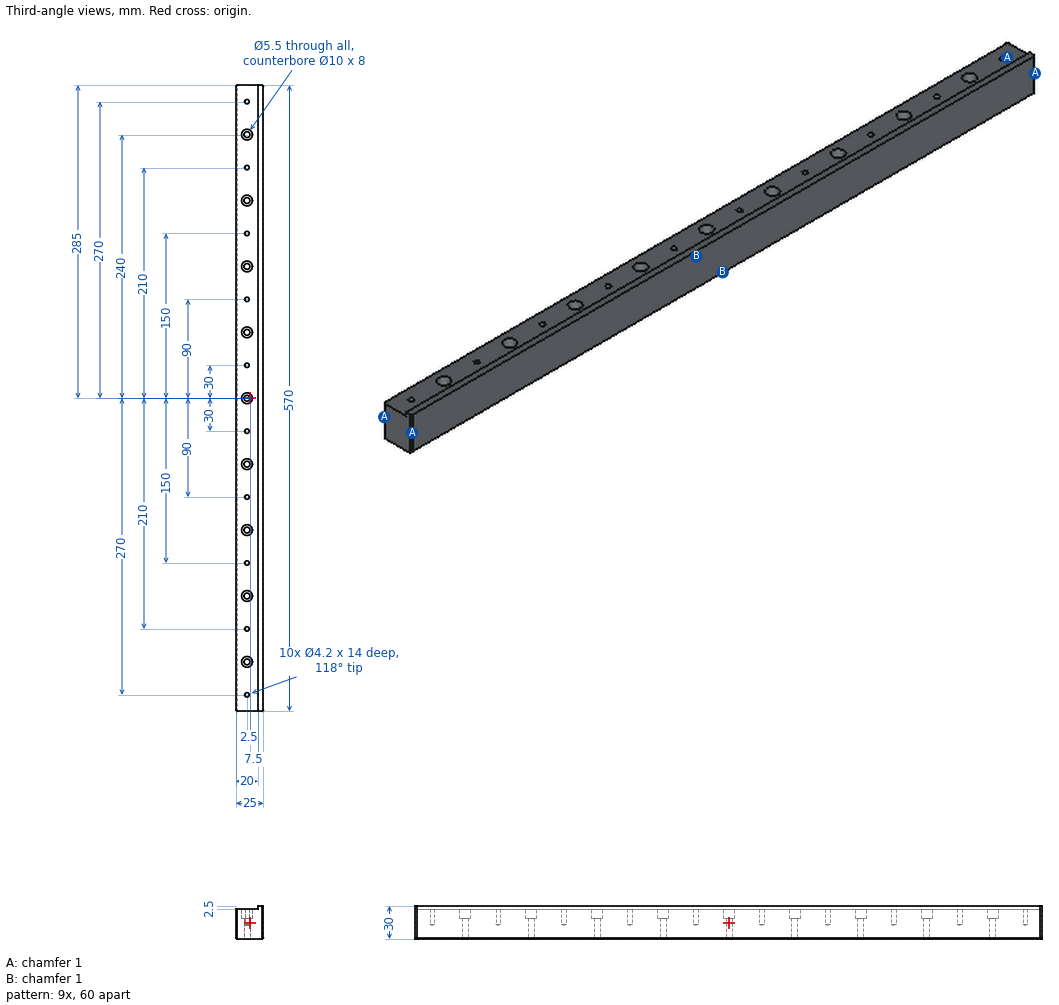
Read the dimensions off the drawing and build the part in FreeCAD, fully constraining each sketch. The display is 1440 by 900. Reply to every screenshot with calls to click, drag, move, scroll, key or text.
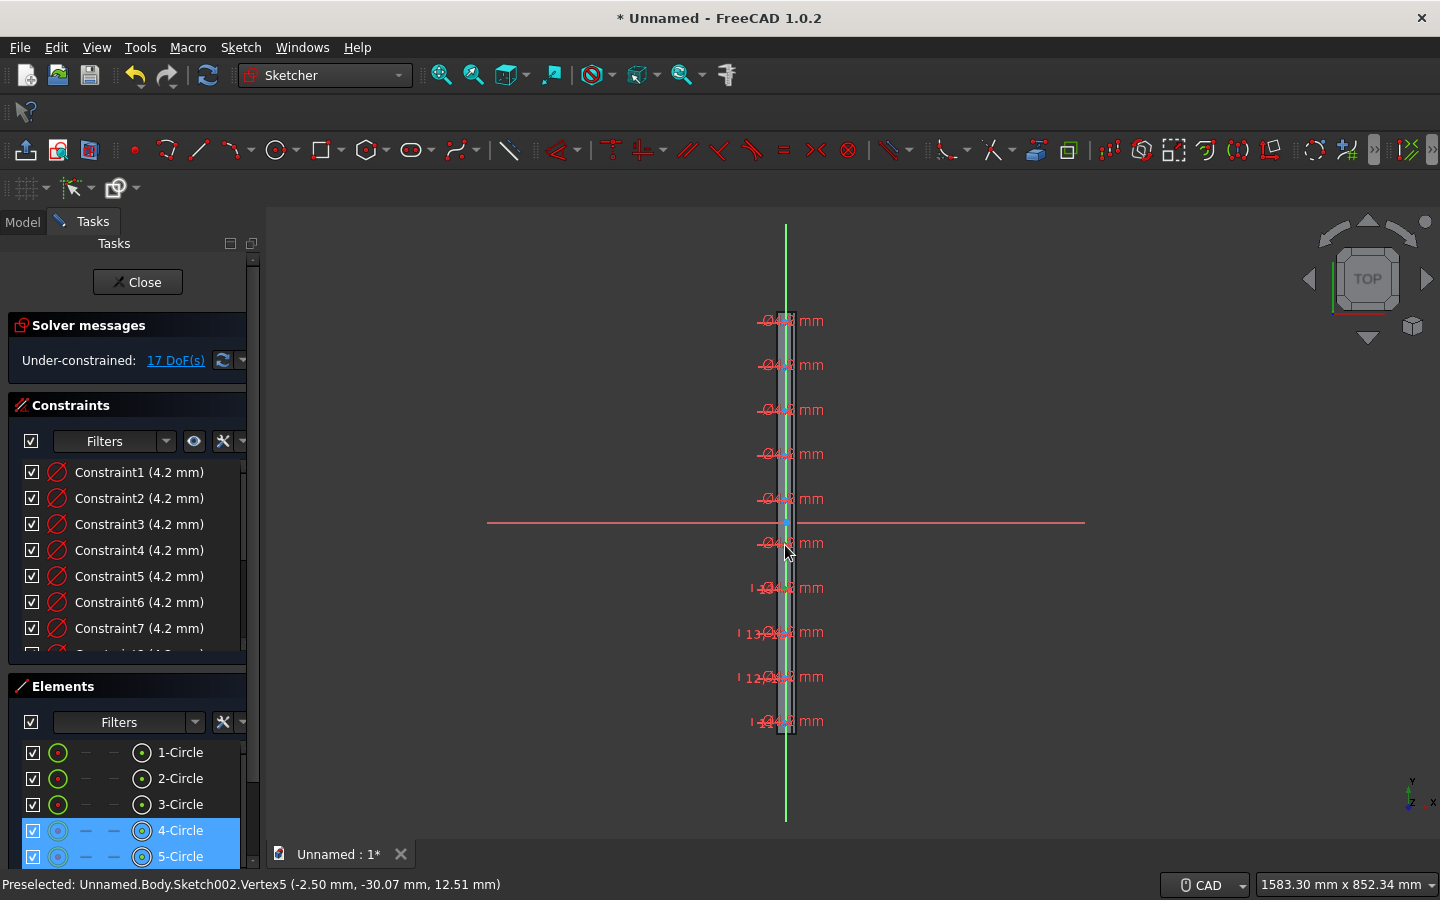
key(v)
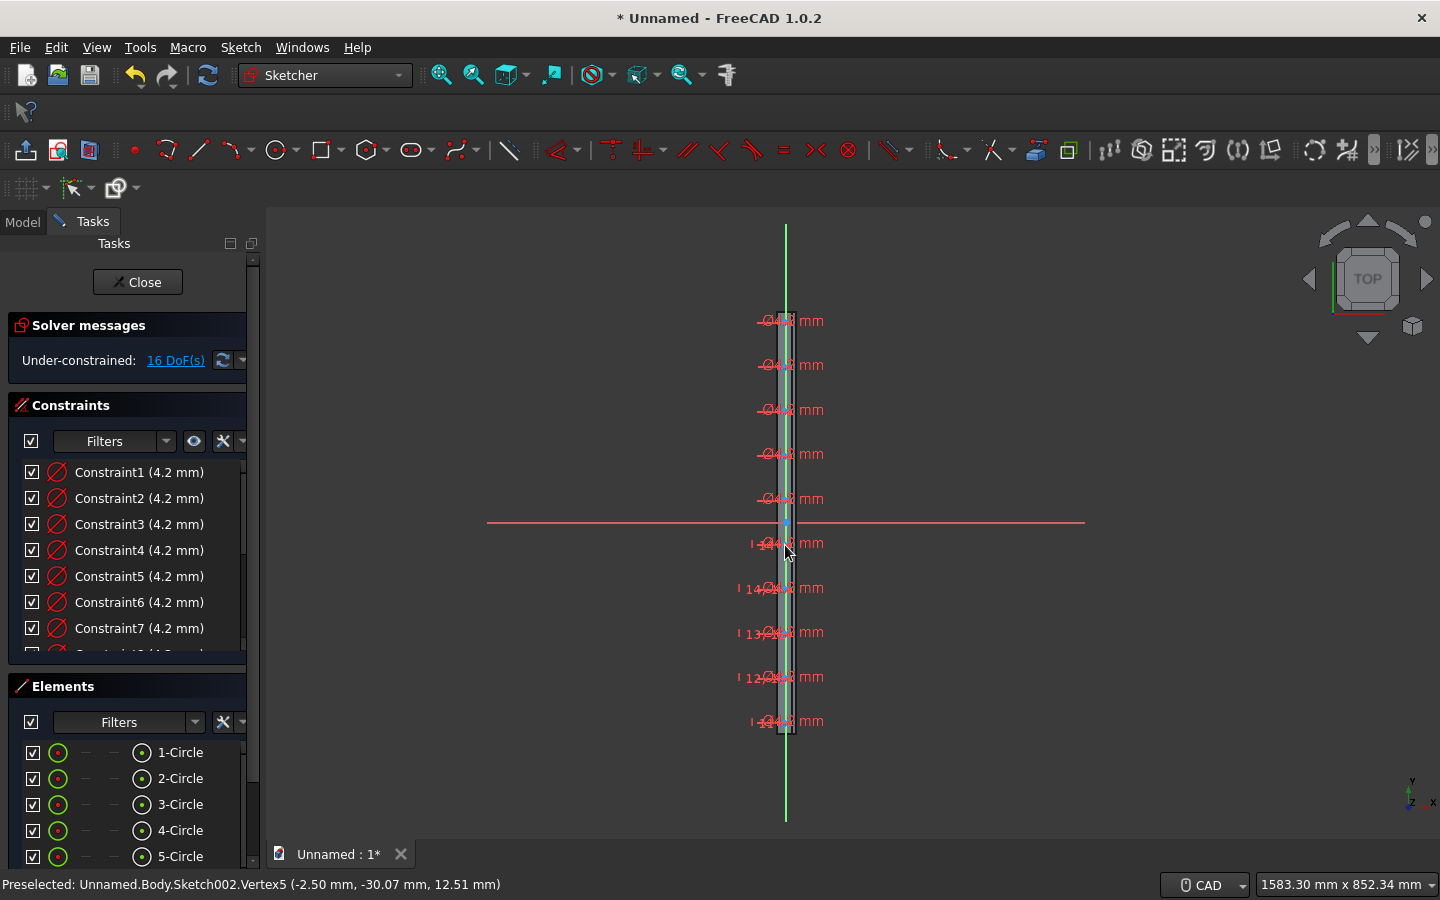
click(785, 545)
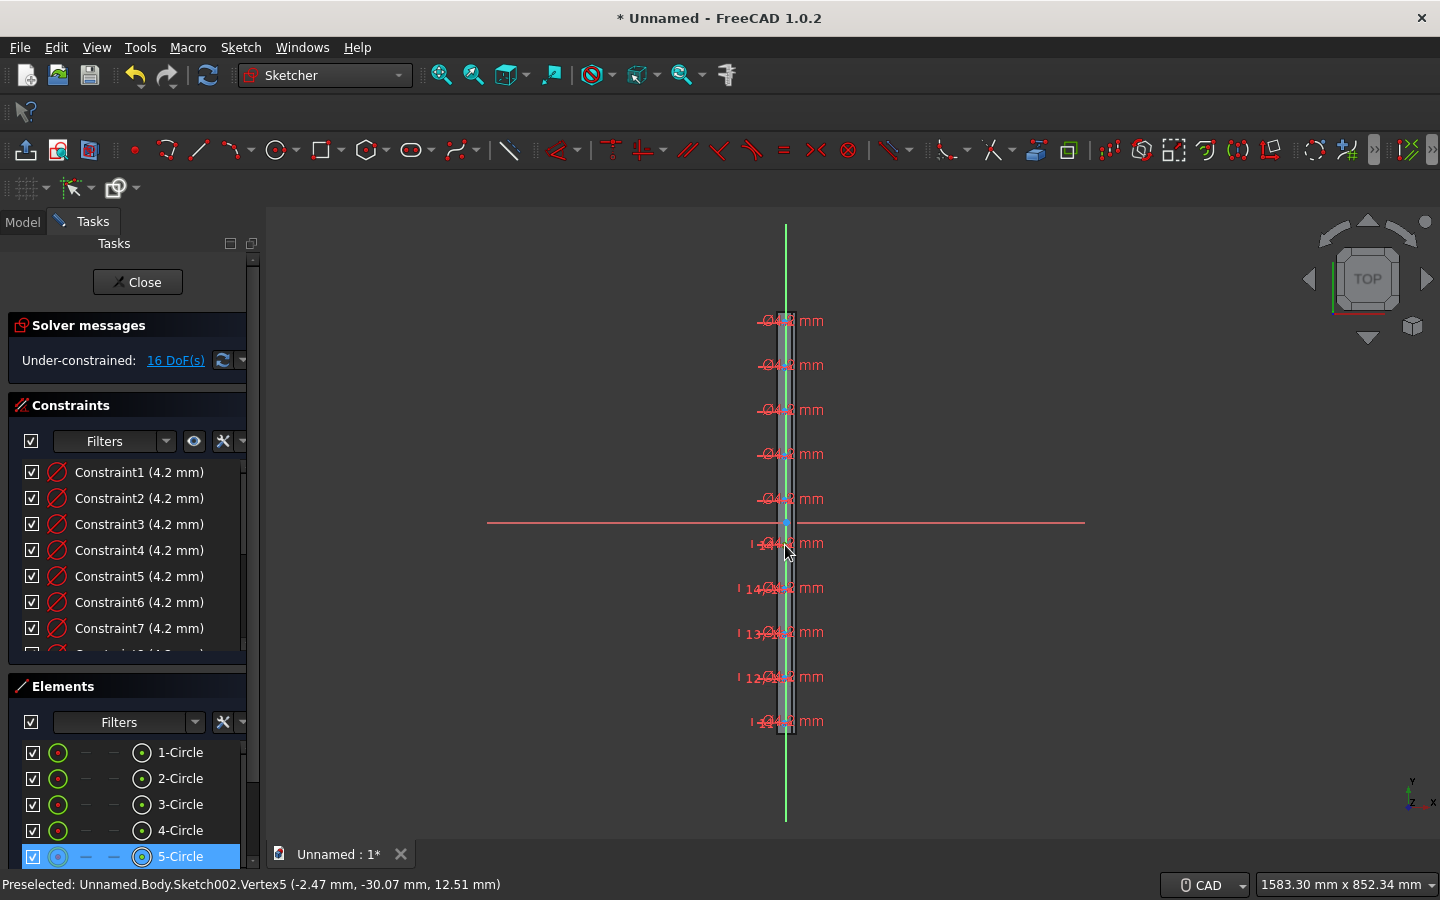
click(785, 501)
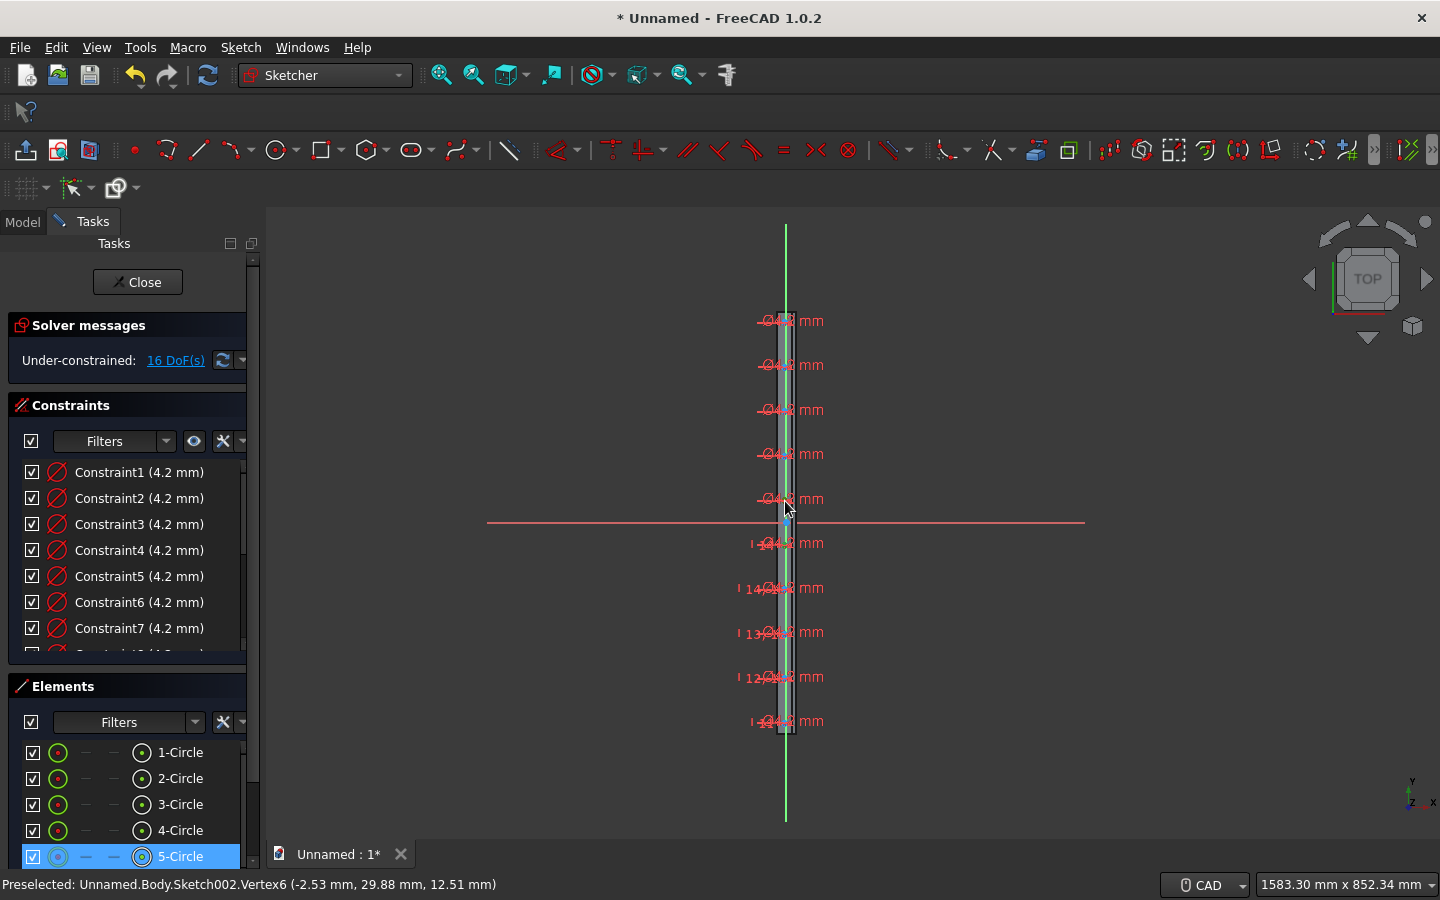
key(v)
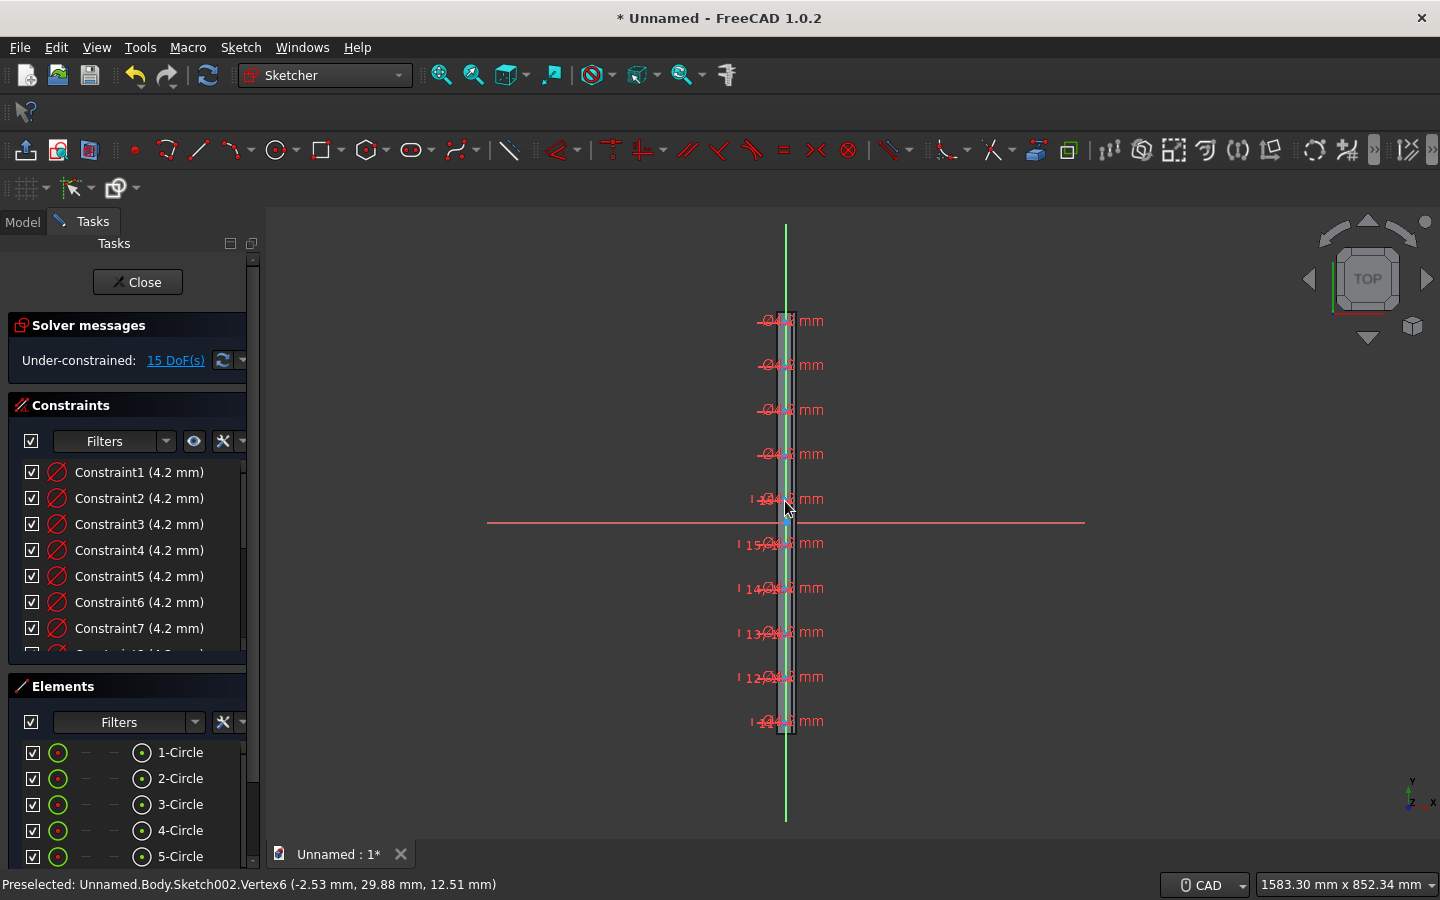
click(785, 501)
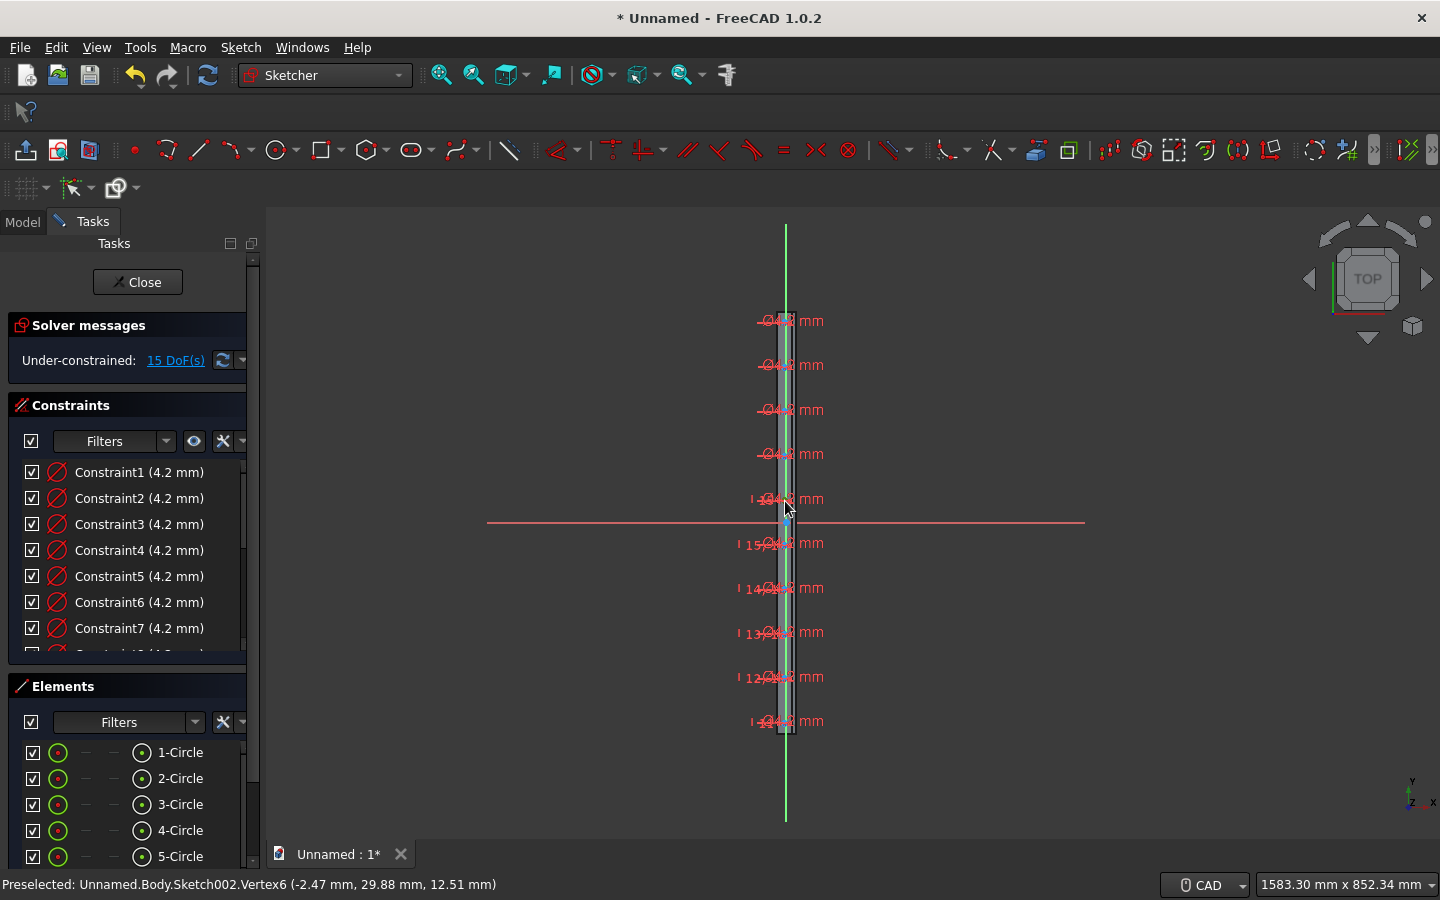
click(785, 456)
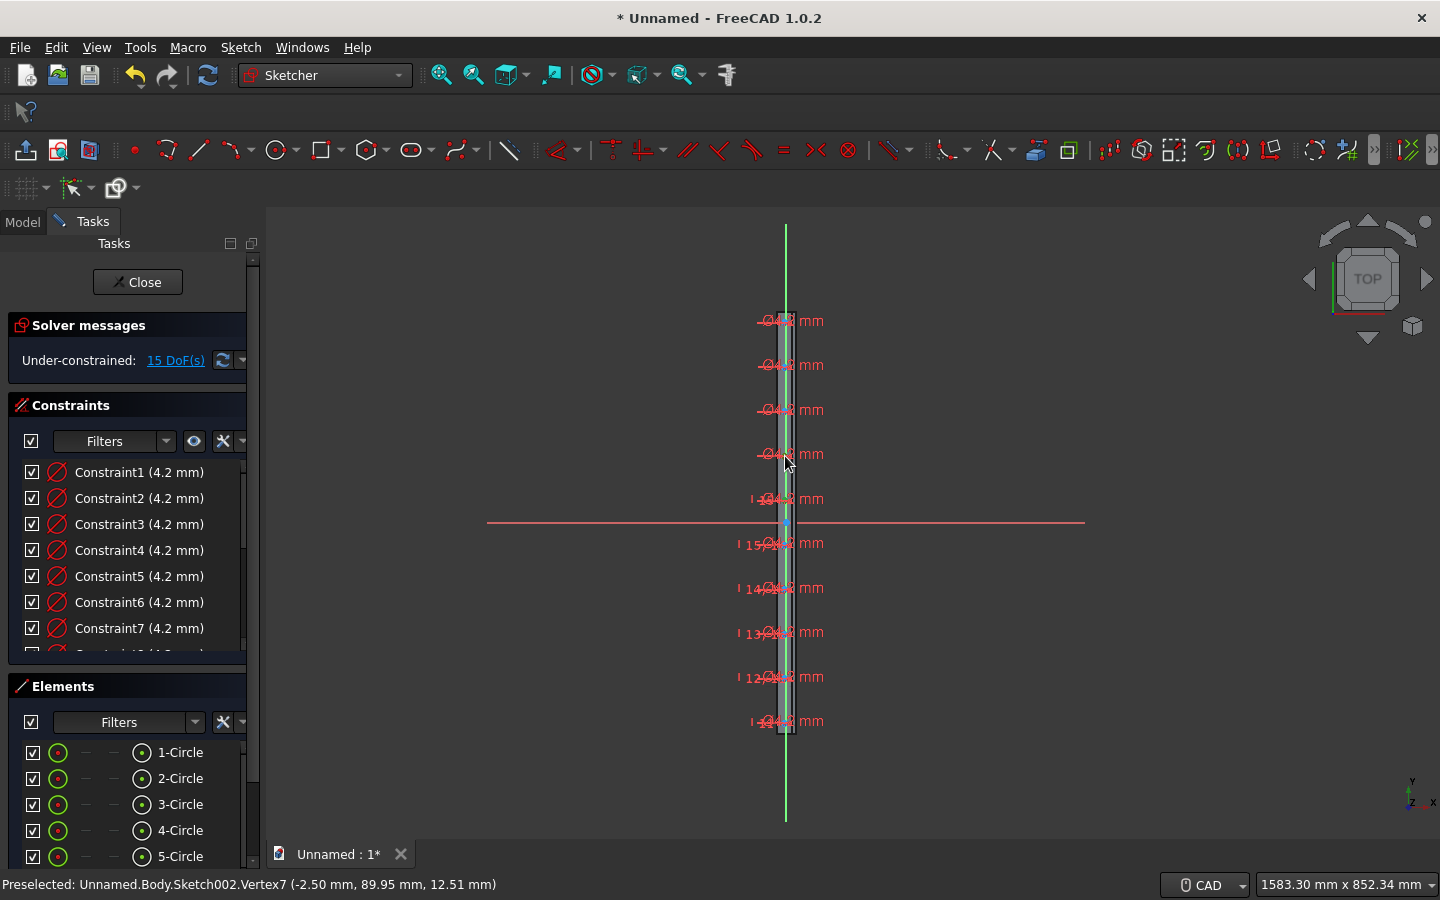
key(v)